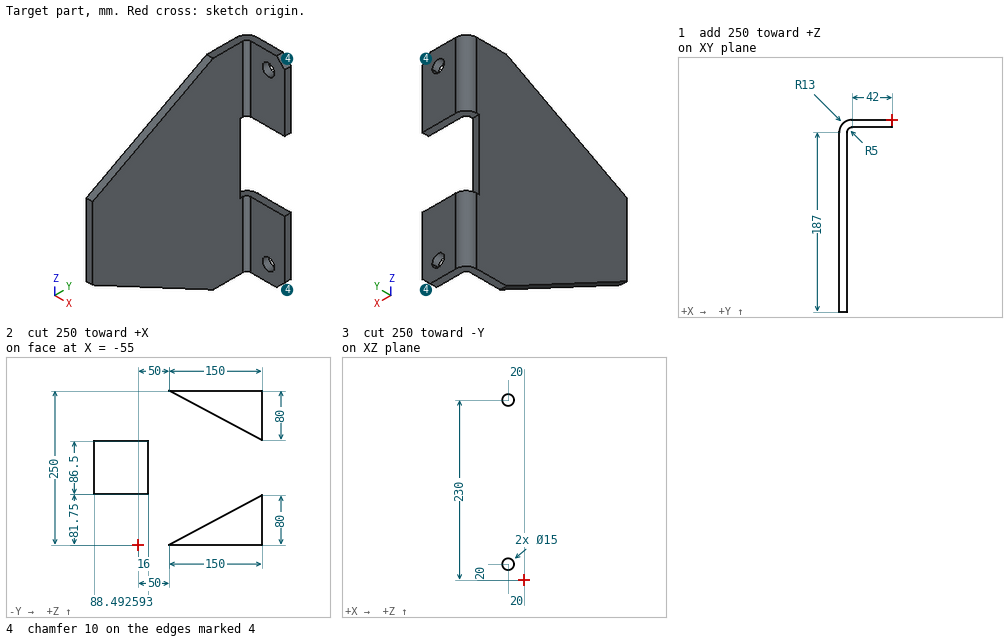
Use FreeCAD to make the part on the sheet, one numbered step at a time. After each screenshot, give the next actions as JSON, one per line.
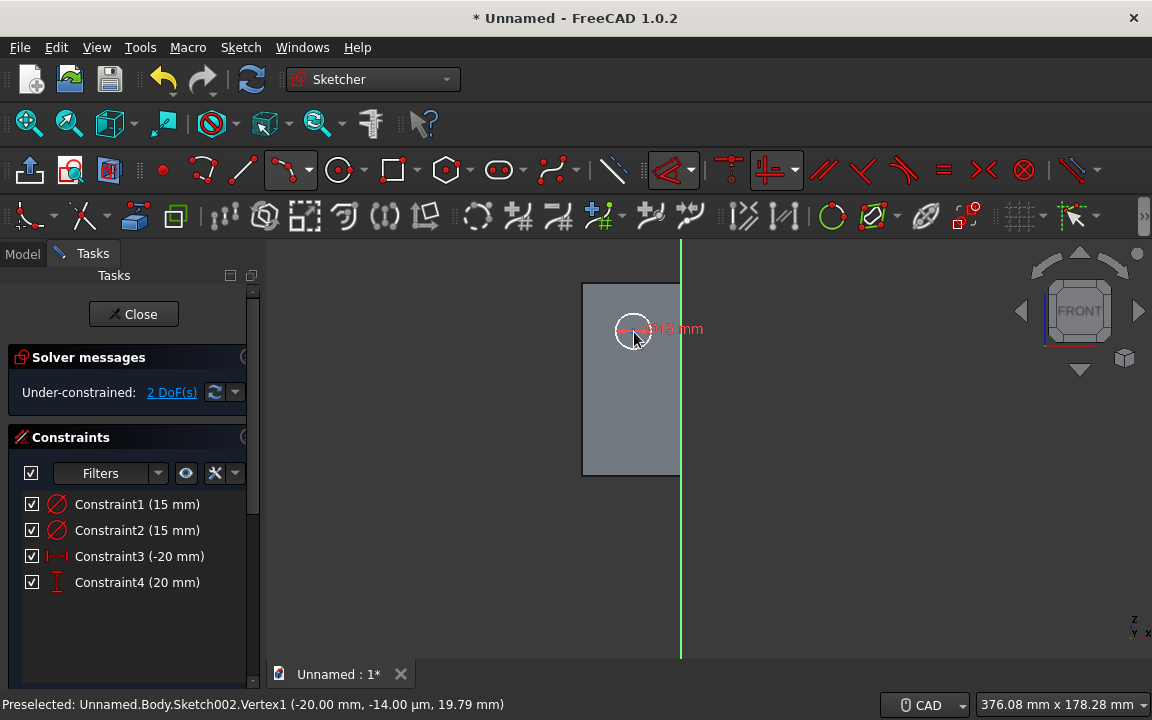
{"action": "left_click", "coordinate": [633, 331]}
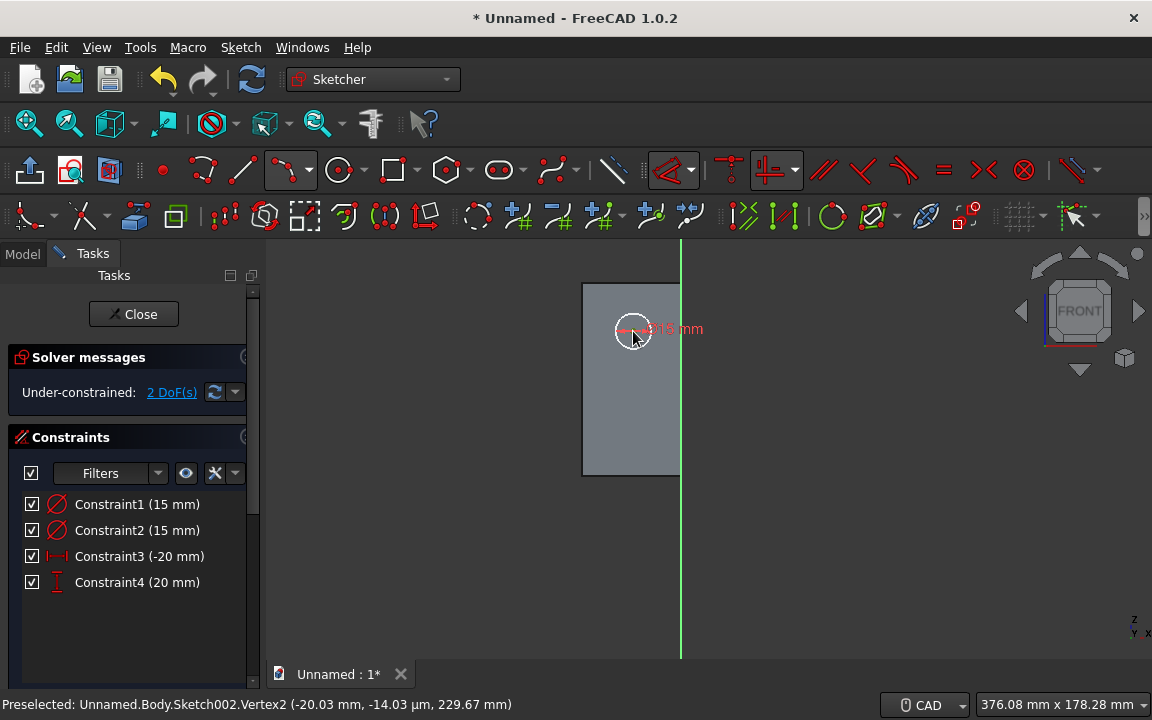
{"action": "left_click", "coordinate": [694, 170]}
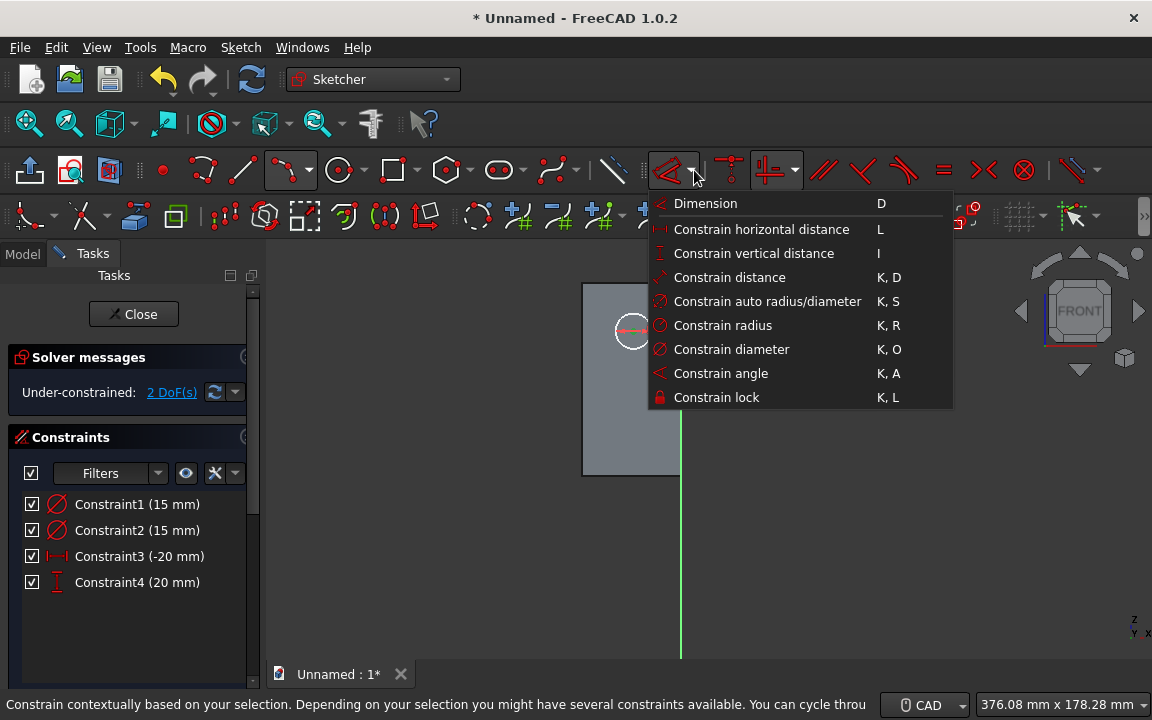
{"action": "left_click", "coordinate": [801, 229]}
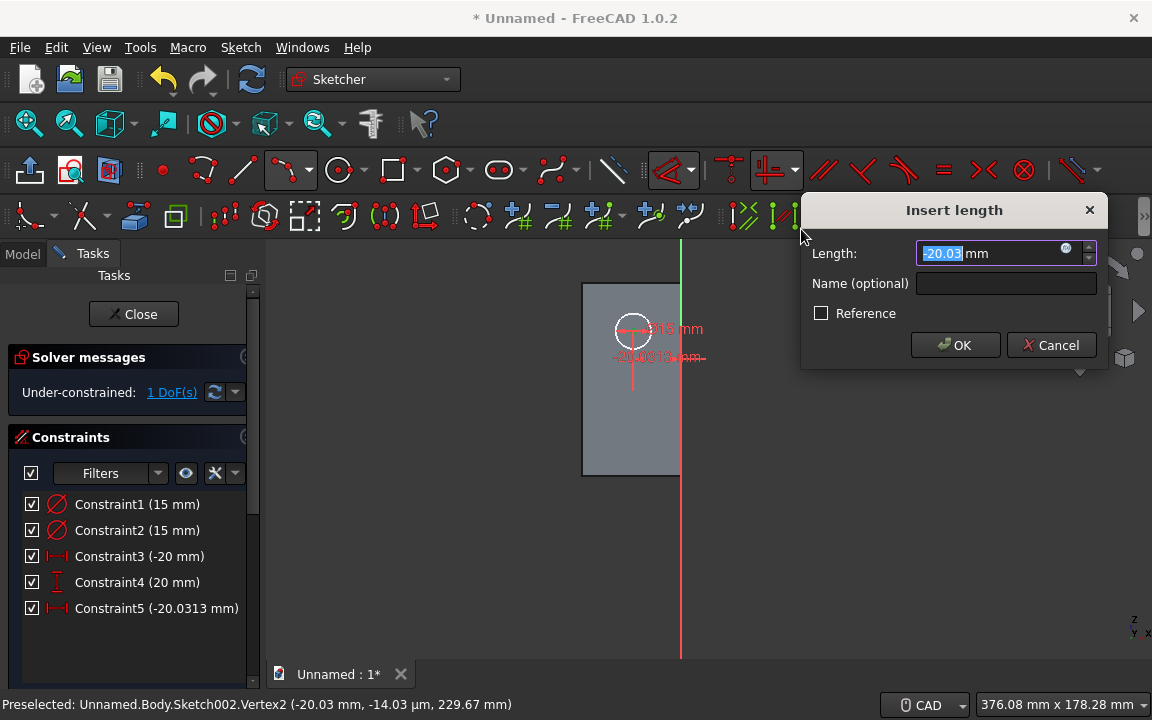
{"action": "type", "text": "-20"}
{"action": "key", "text": "Return"}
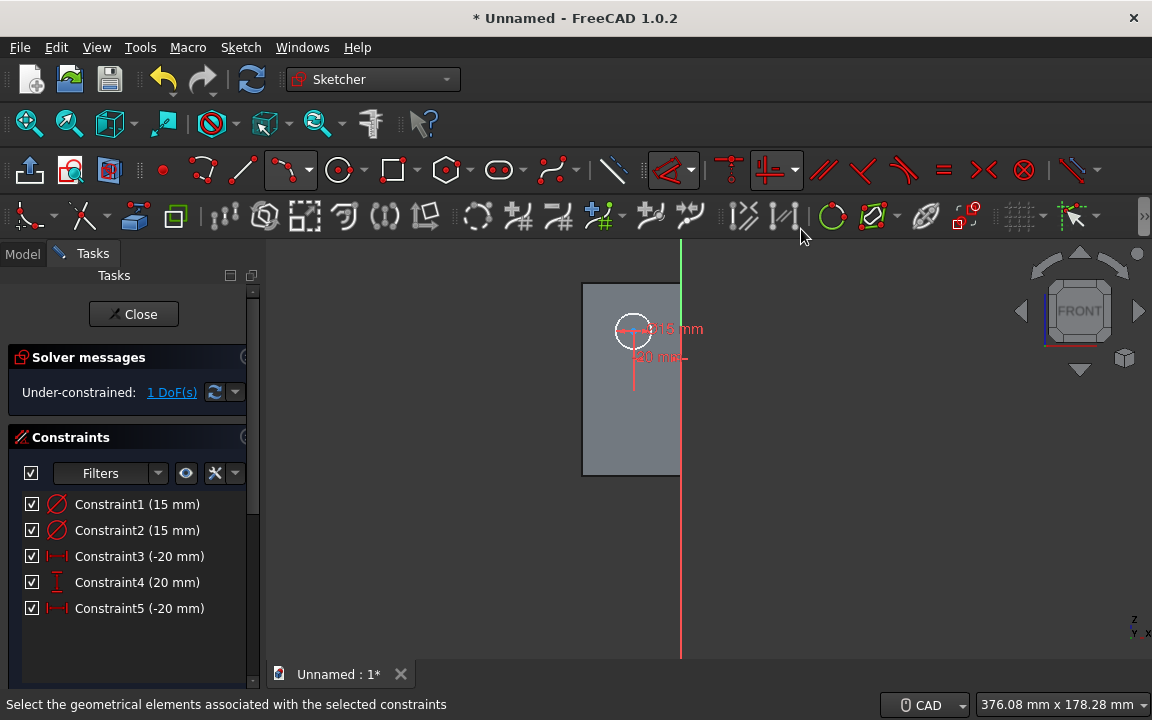
{"action": "left_click", "coordinate": [634, 331]}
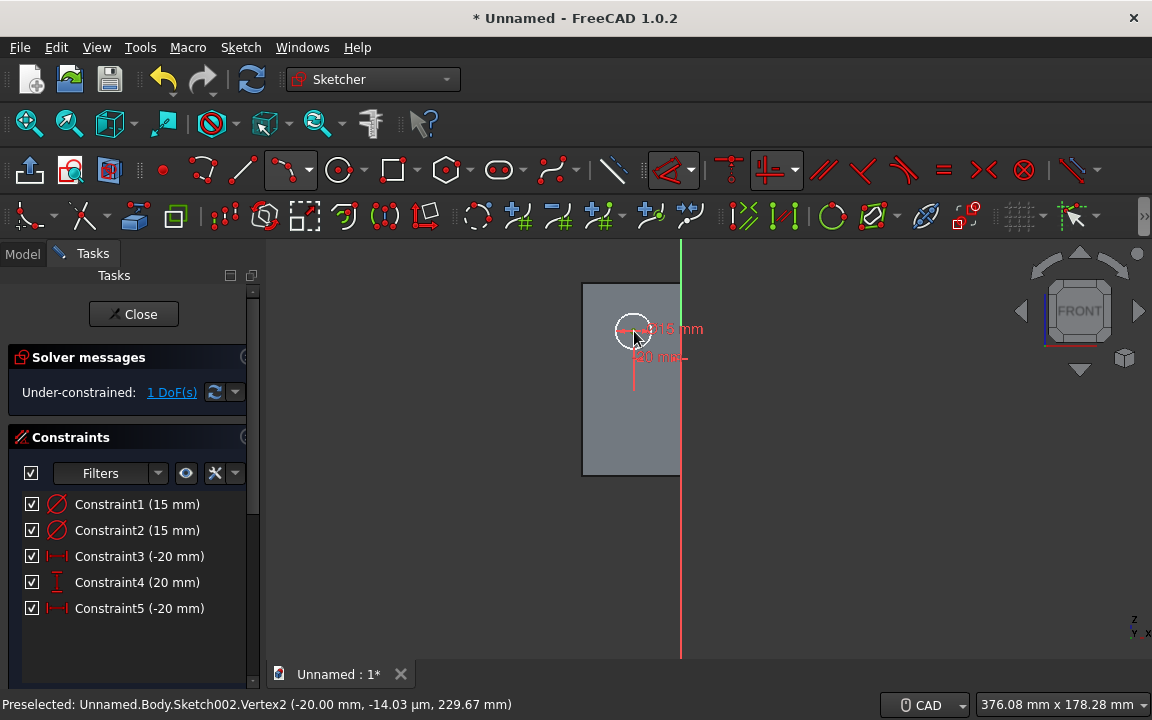
{"action": "key", "text": "i"}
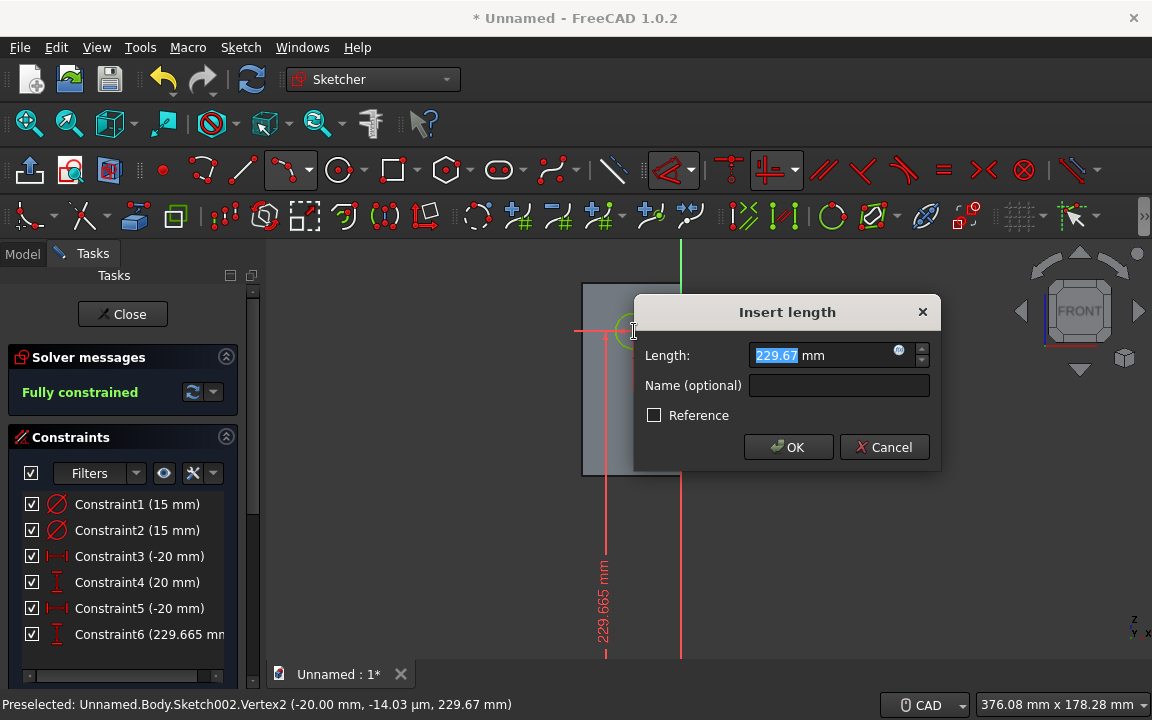
{"action": "type", "text": "230"}
{"action": "key", "text": "Return"}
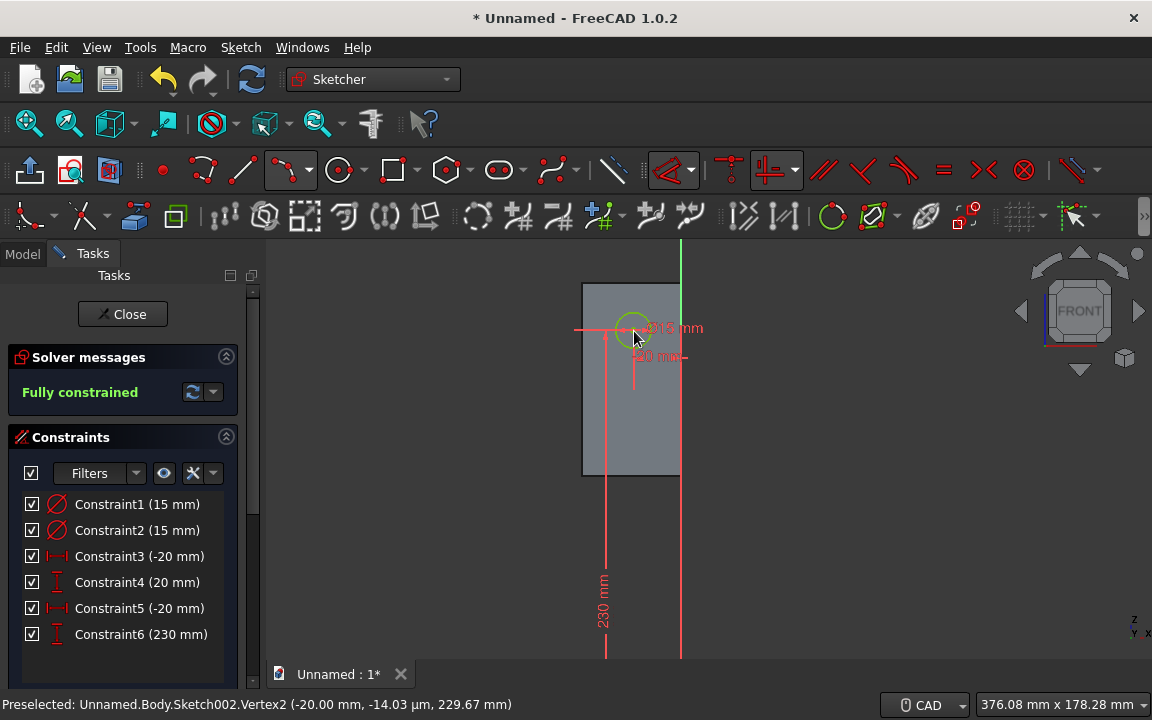
{"action": "left_click", "coordinate": [123, 314]}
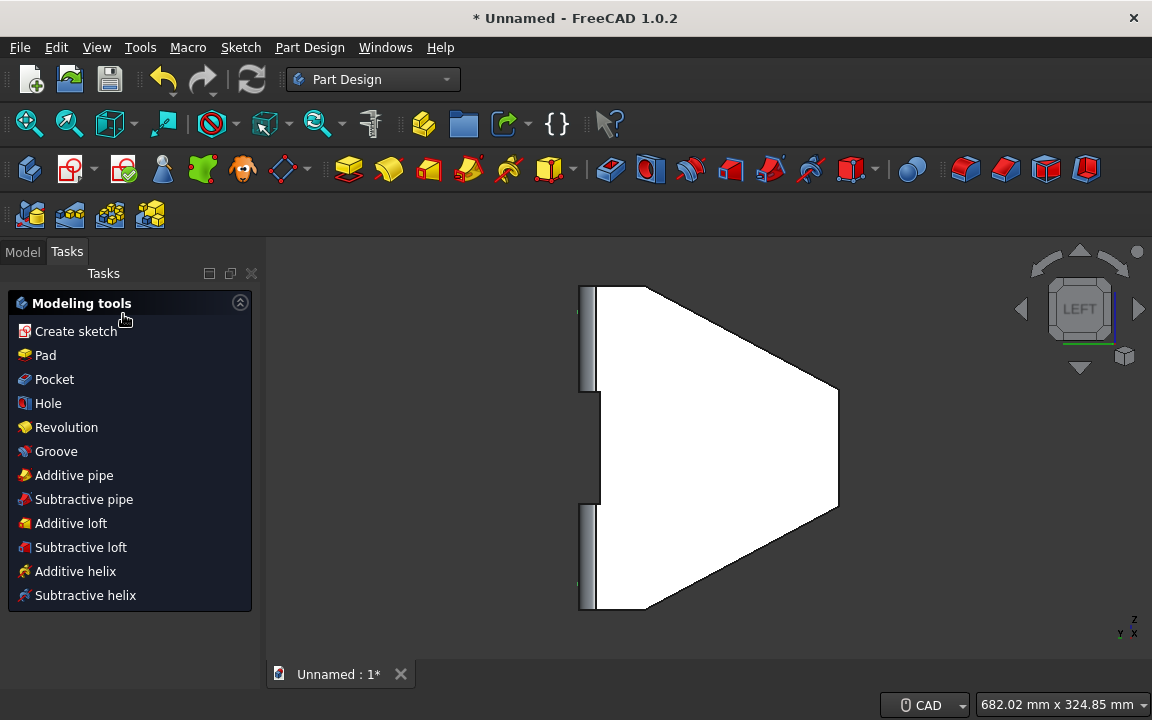
{"action": "left_click", "coordinate": [612, 170]}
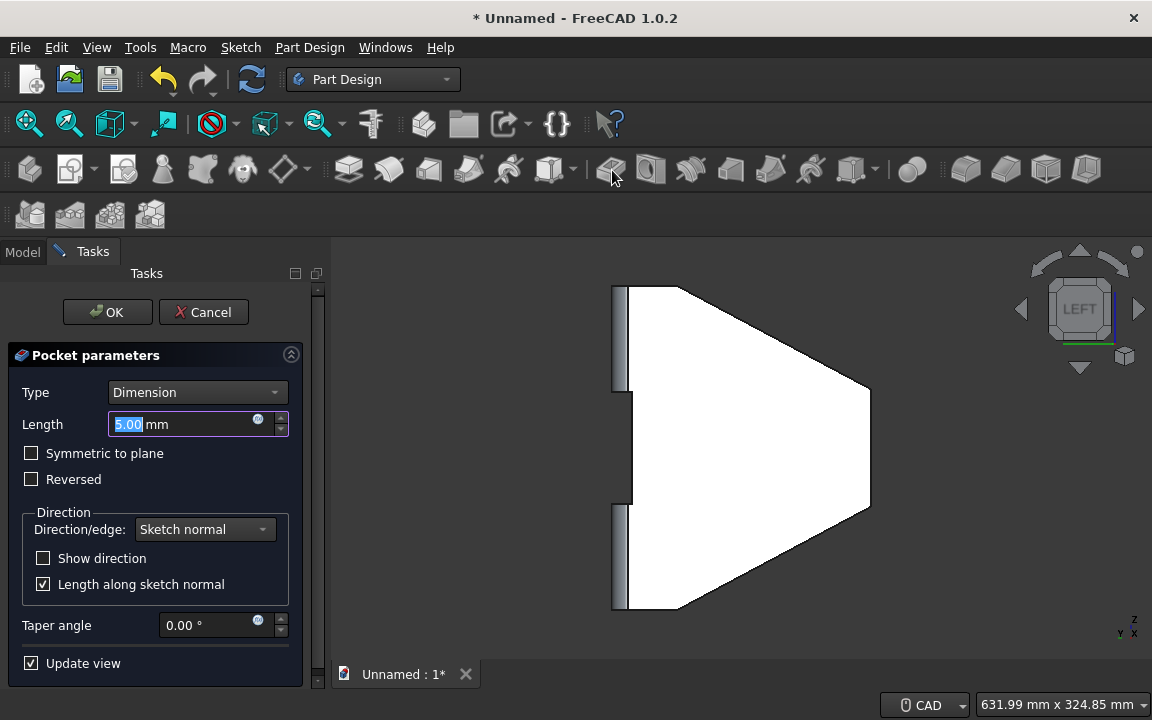
{"action": "type", "text": "250"}
{"action": "key", "text": "Tab"}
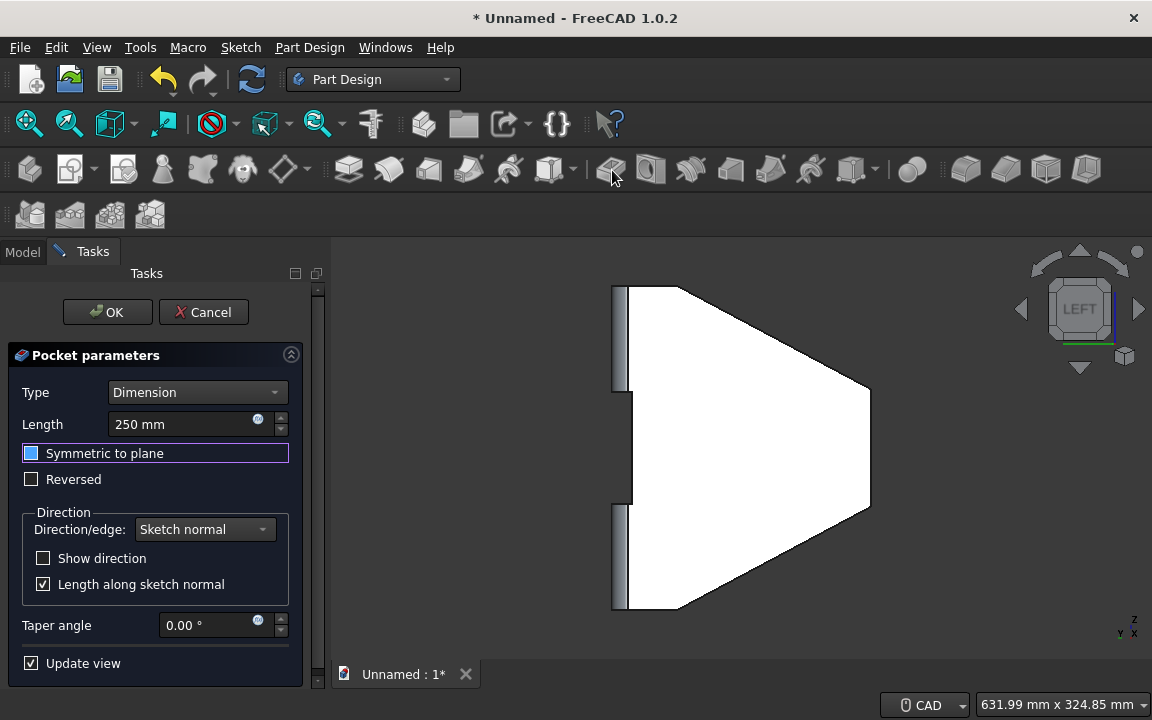
{"action": "left_click", "coordinate": [30, 479]}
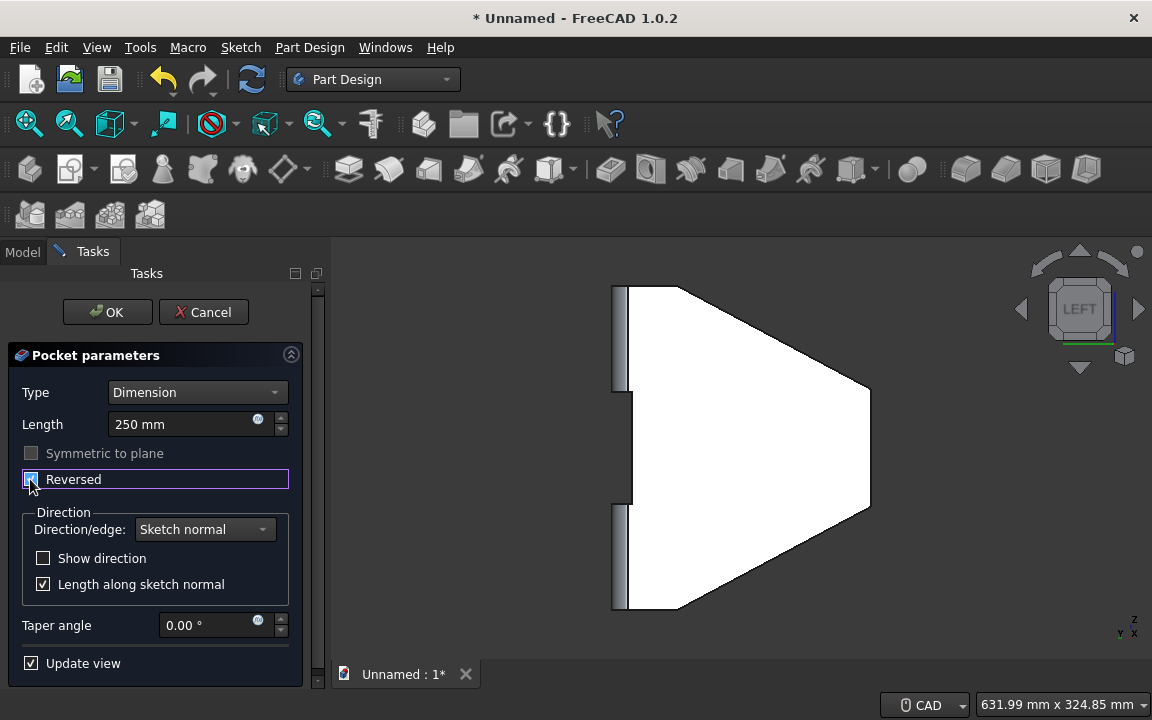
{"action": "left_click", "coordinate": [108, 312]}